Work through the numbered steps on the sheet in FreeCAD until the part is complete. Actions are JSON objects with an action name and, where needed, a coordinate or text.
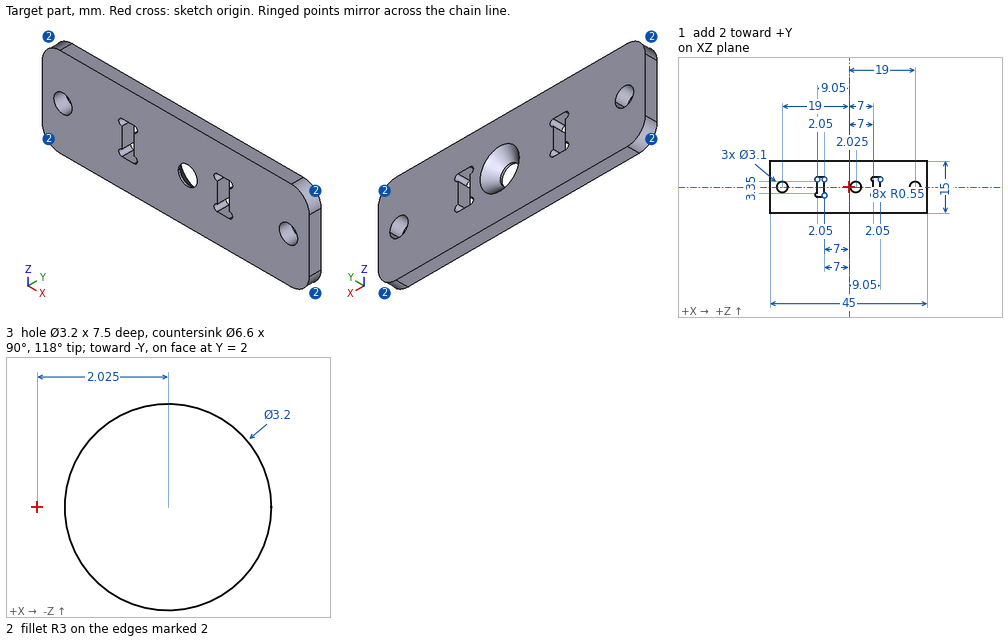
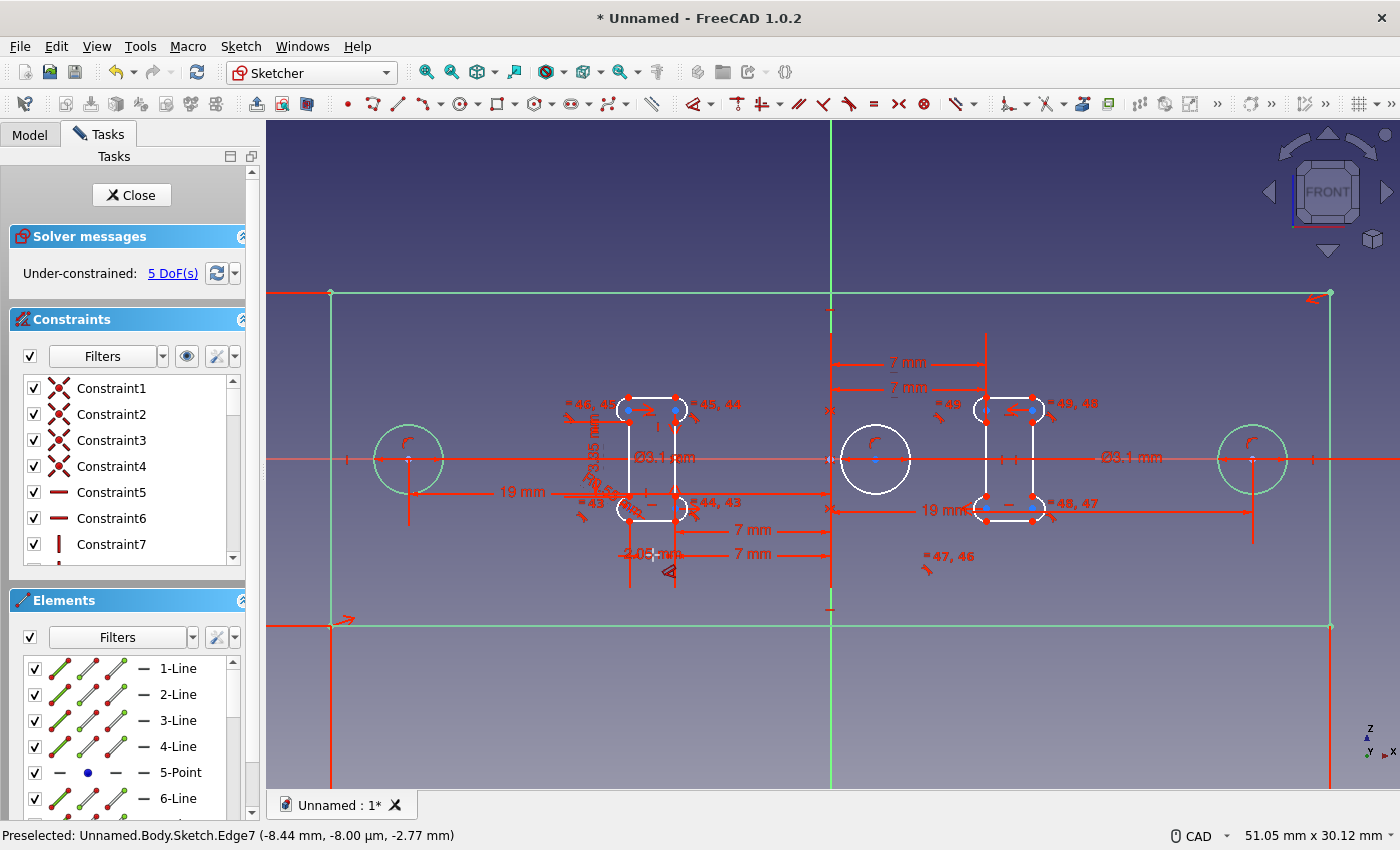
{"action": "left_click", "coordinate": [661, 398]}
{"action": "left_click", "coordinate": [652, 364]}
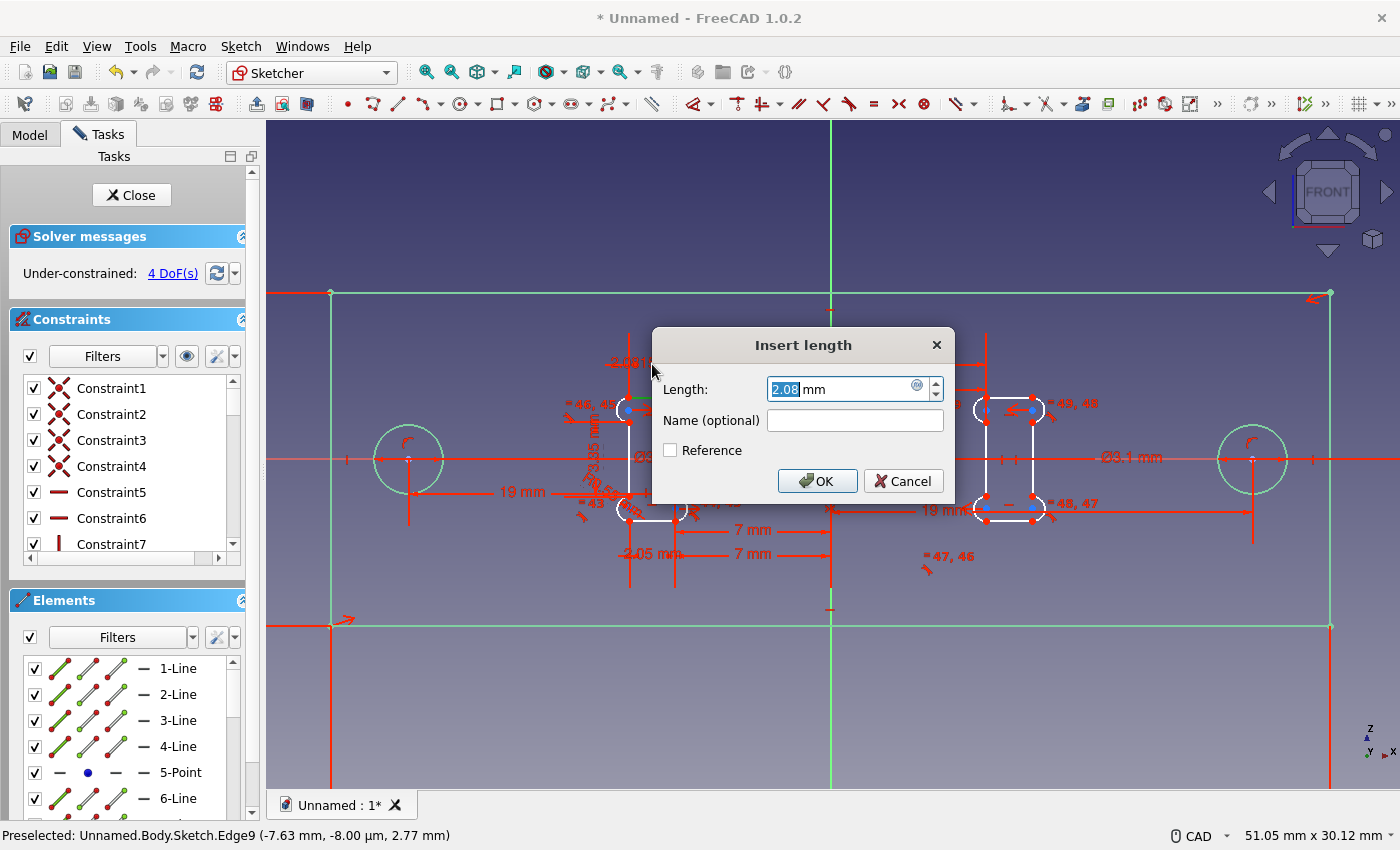
{"action": "type", "text": "2.05"}
{"action": "key", "text": "Return"}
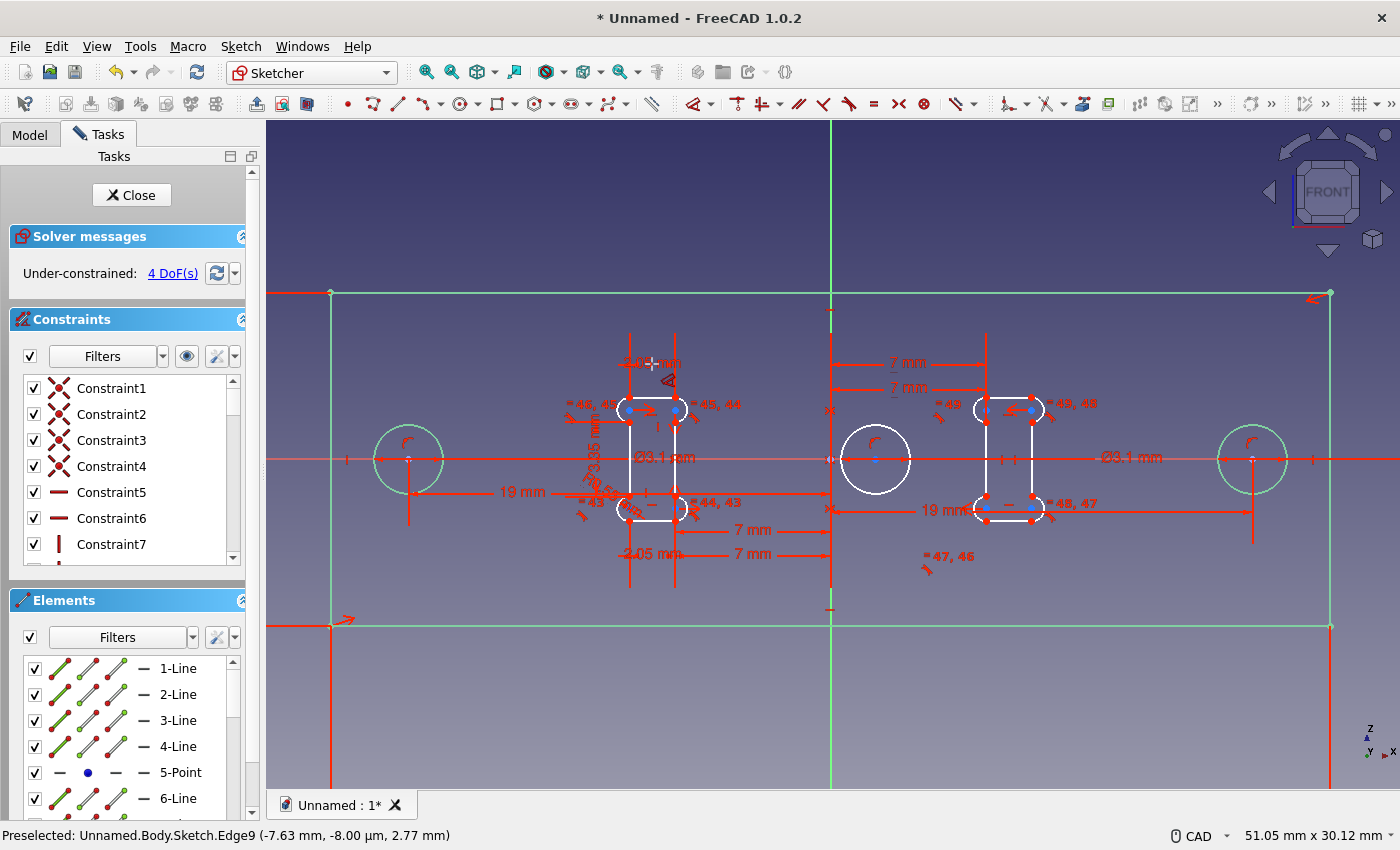
{"action": "left_click", "coordinate": [1000, 521]}
{"action": "left_click", "coordinate": [1009, 555]}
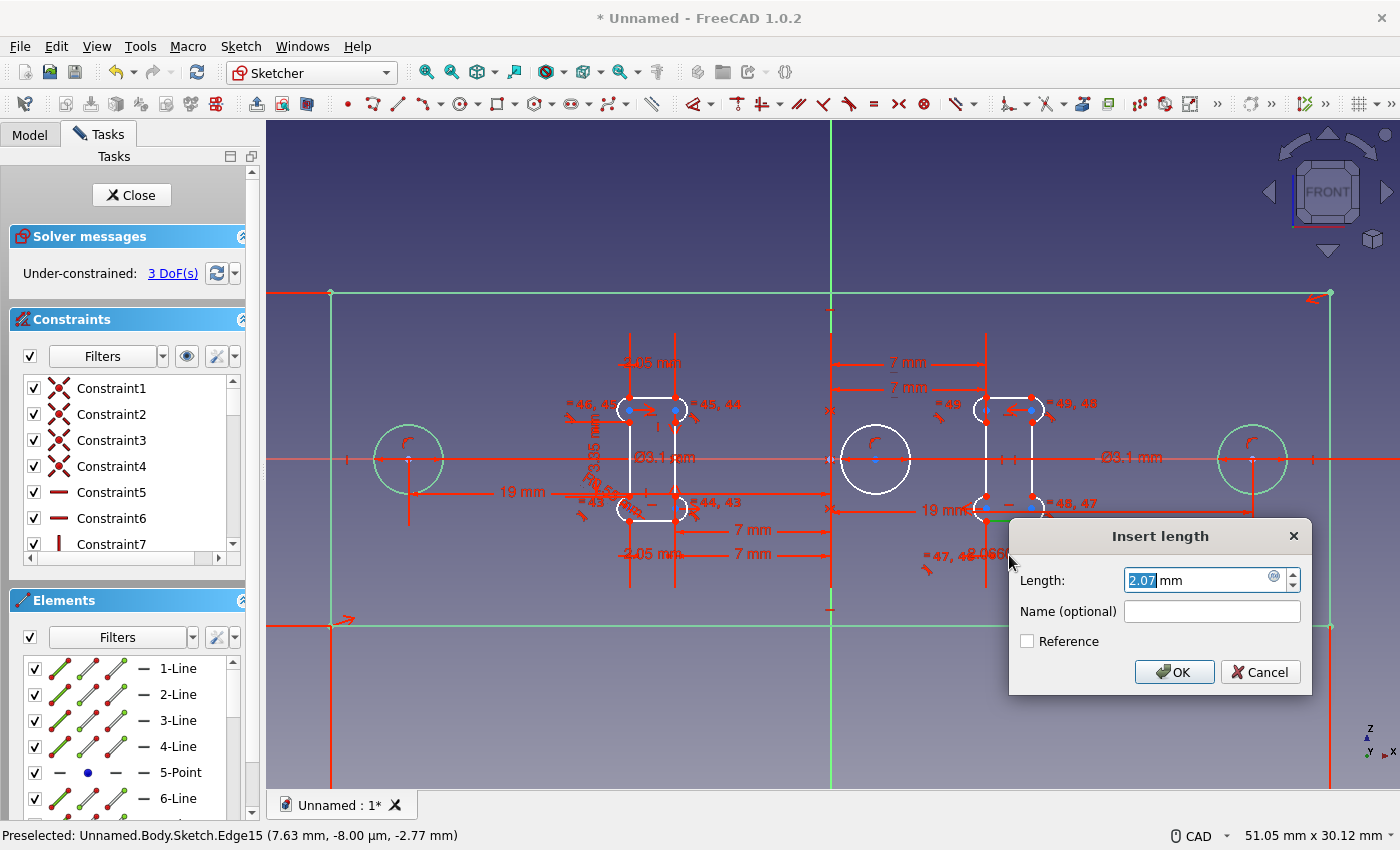
{"action": "type", "text": "2.05"}
{"action": "key", "text": "Return"}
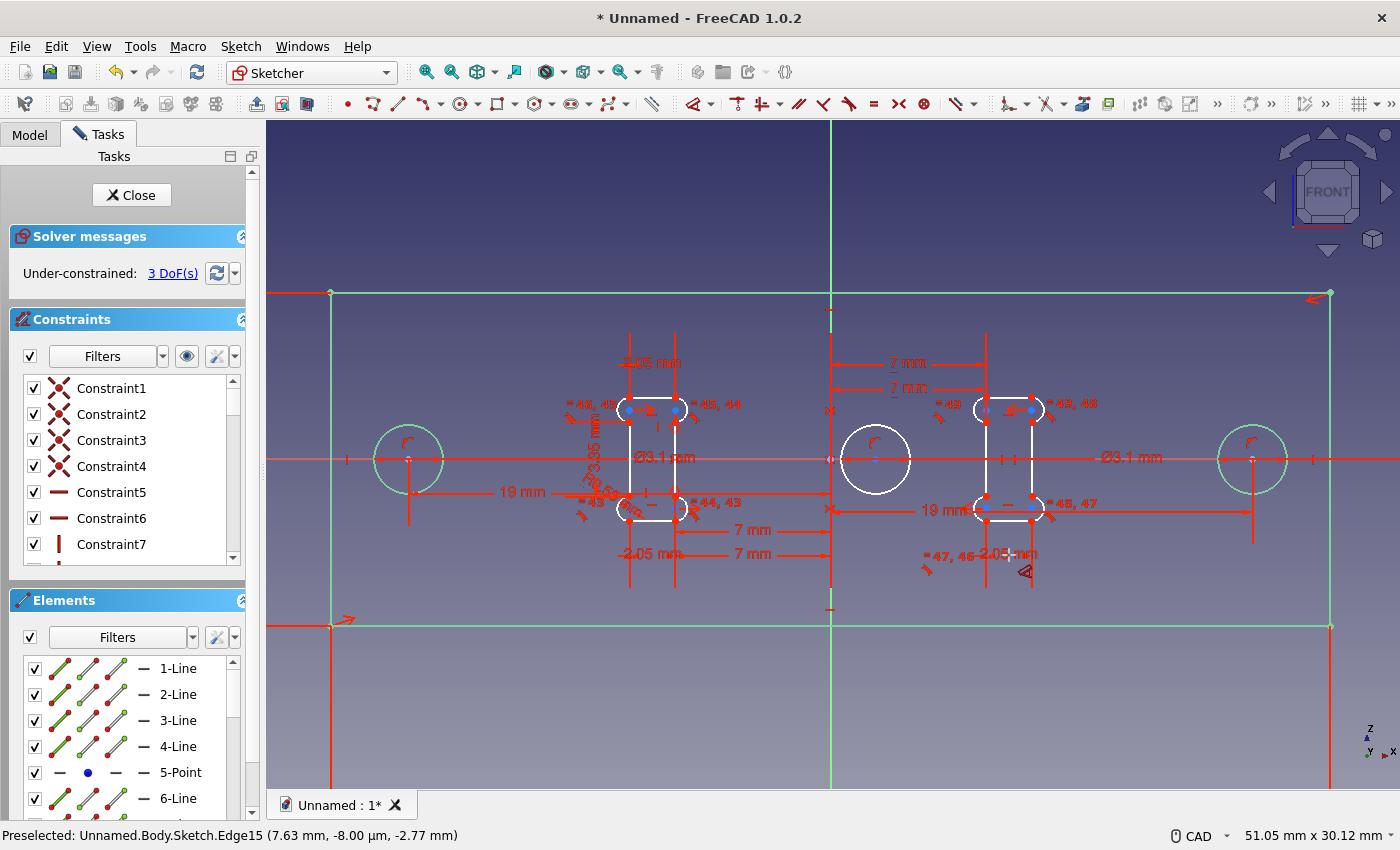
{"action": "left_click", "coordinate": [630, 422]}
{"action": "left_click", "coordinate": [730, 388]}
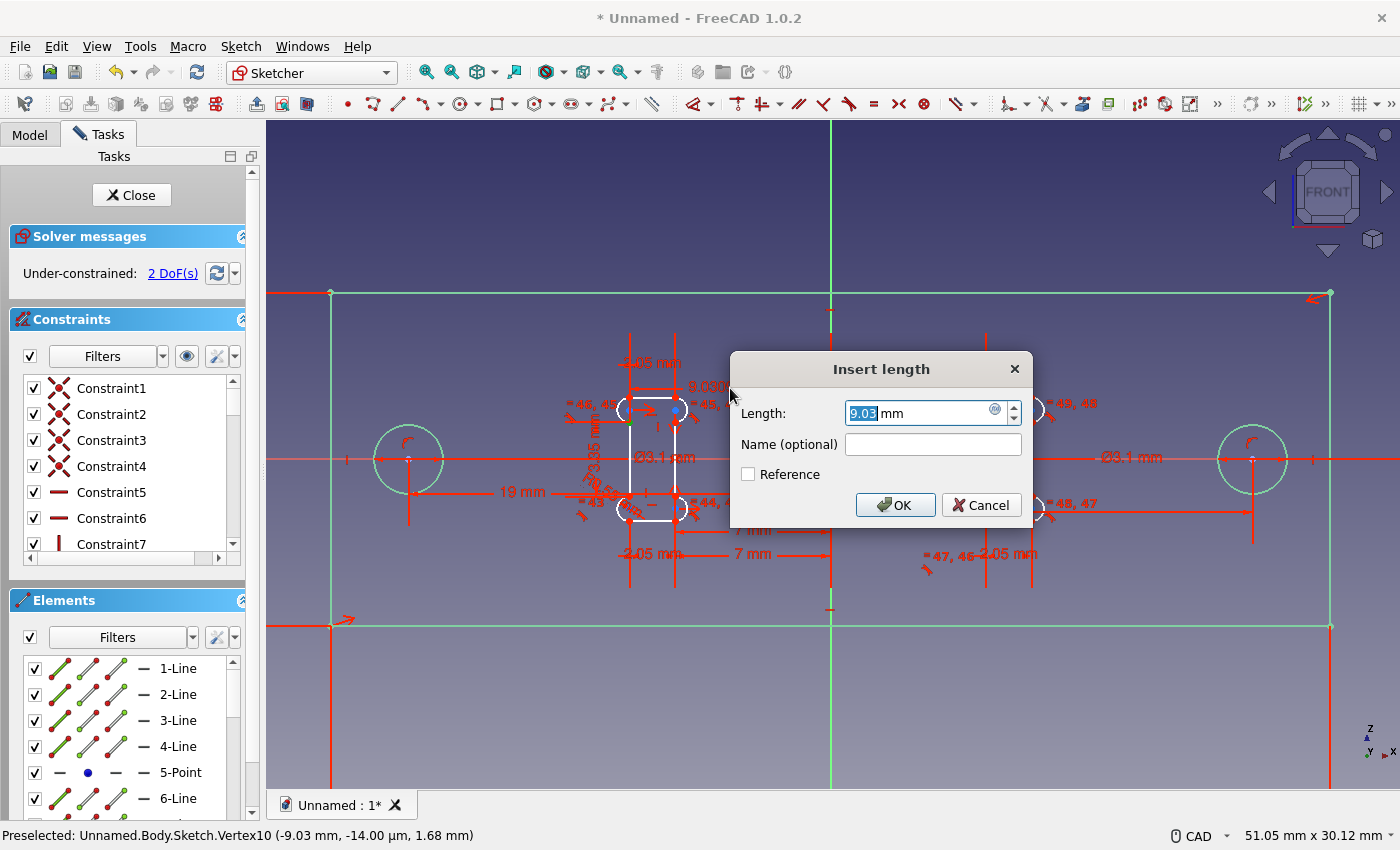
{"action": "type", "text": "9.05"}
{"action": "key", "text": "Return"}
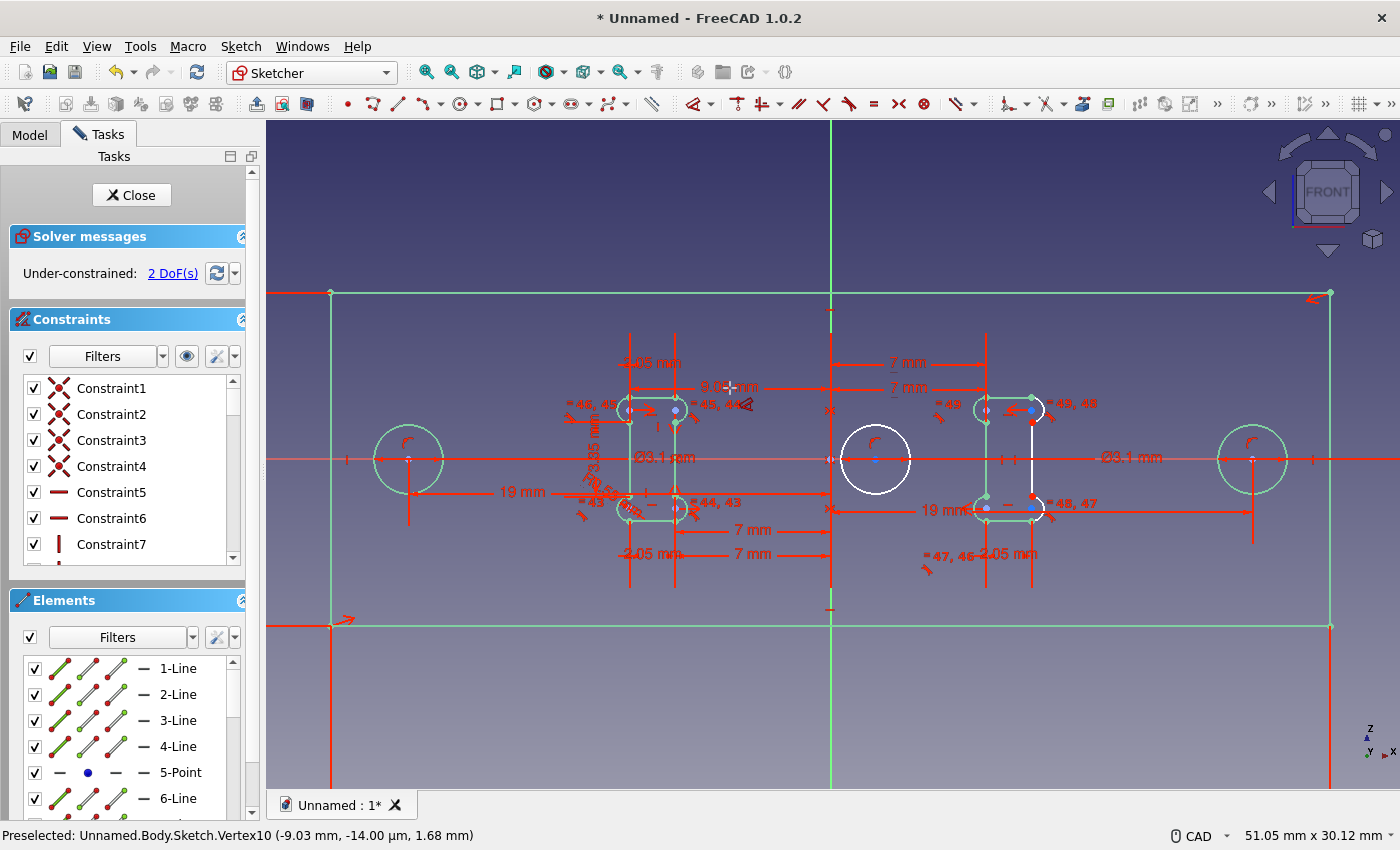
{"action": "left_click", "coordinate": [1032, 497]}
{"action": "left_click", "coordinate": [931, 531]}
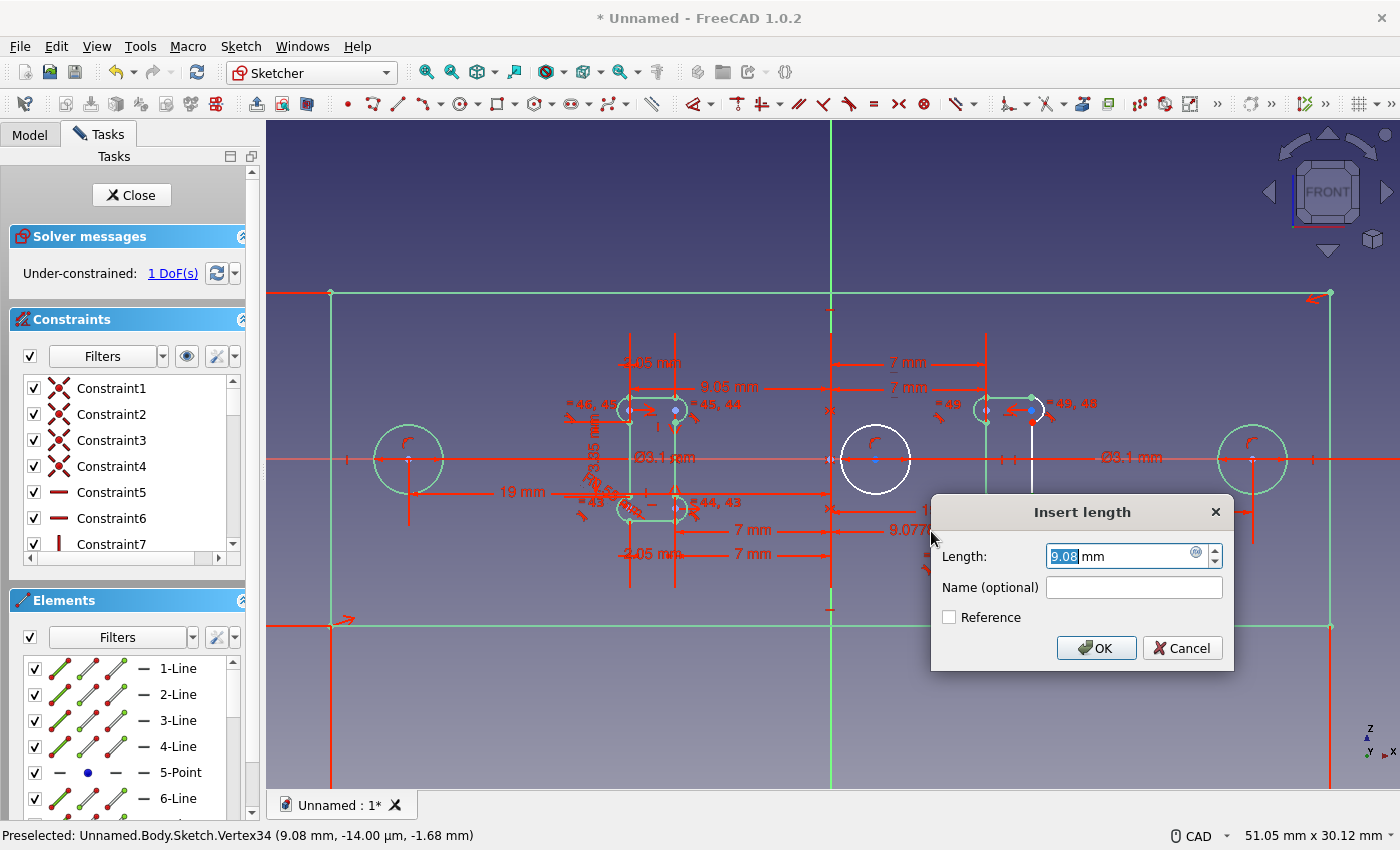
{"action": "type", "text": "9.05"}
{"action": "key", "text": "Return"}